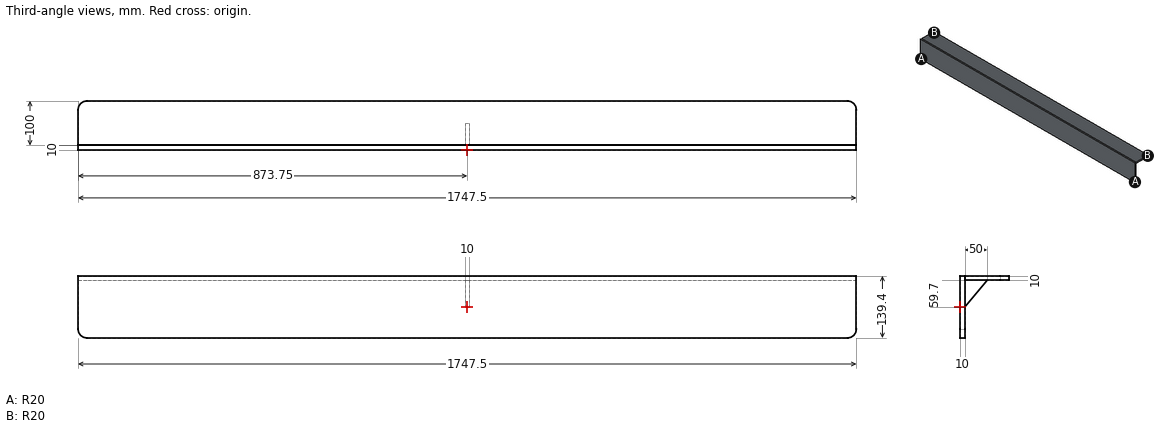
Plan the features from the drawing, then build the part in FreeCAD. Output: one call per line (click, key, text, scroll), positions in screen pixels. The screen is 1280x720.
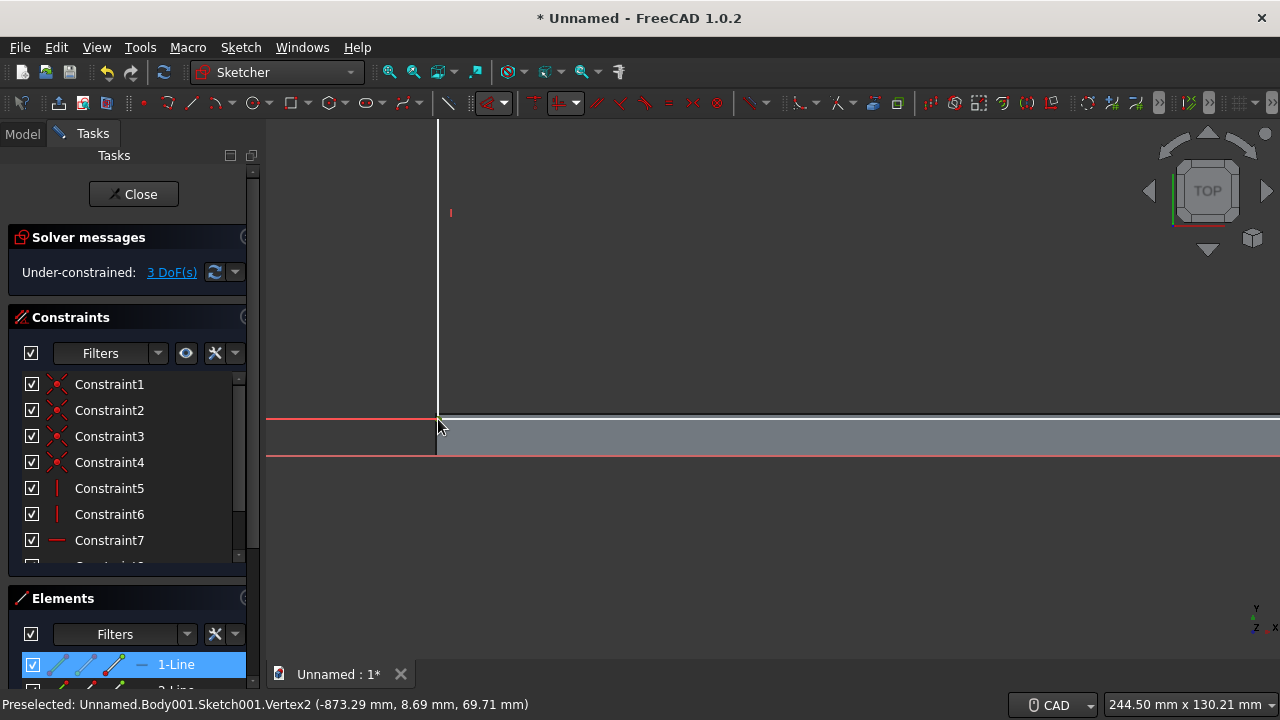
key(i)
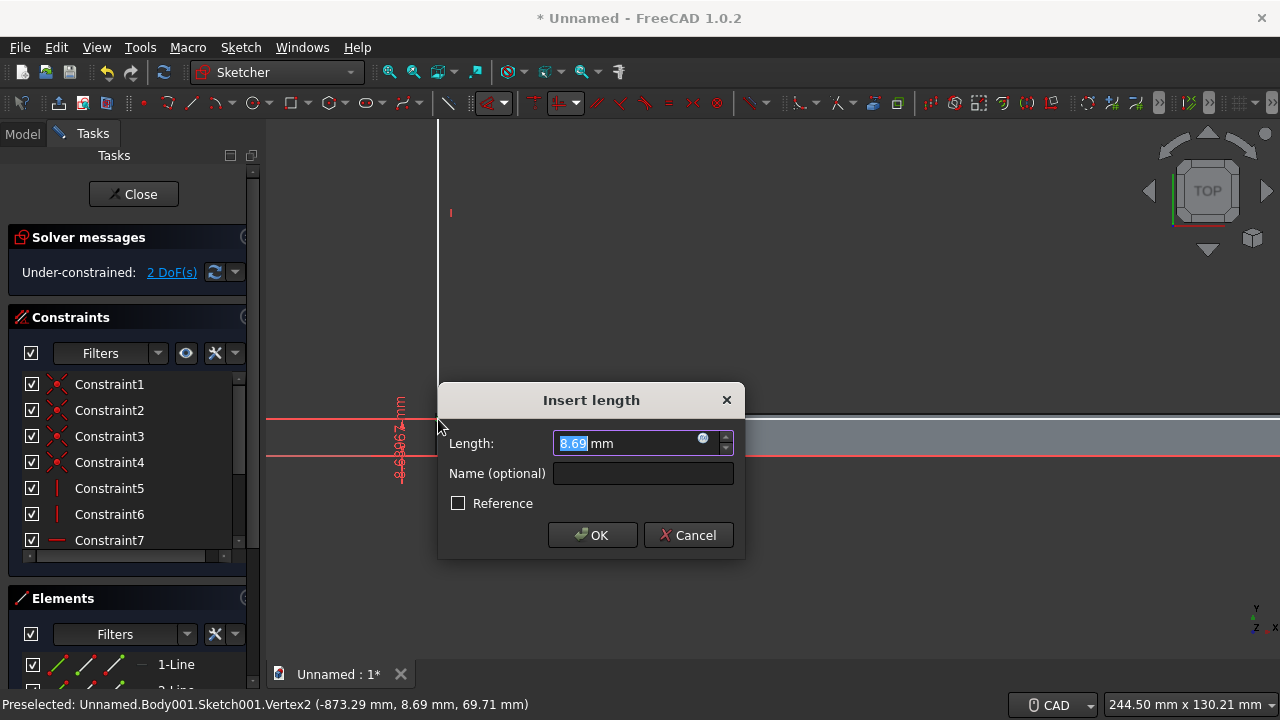
text(10)
key(Return)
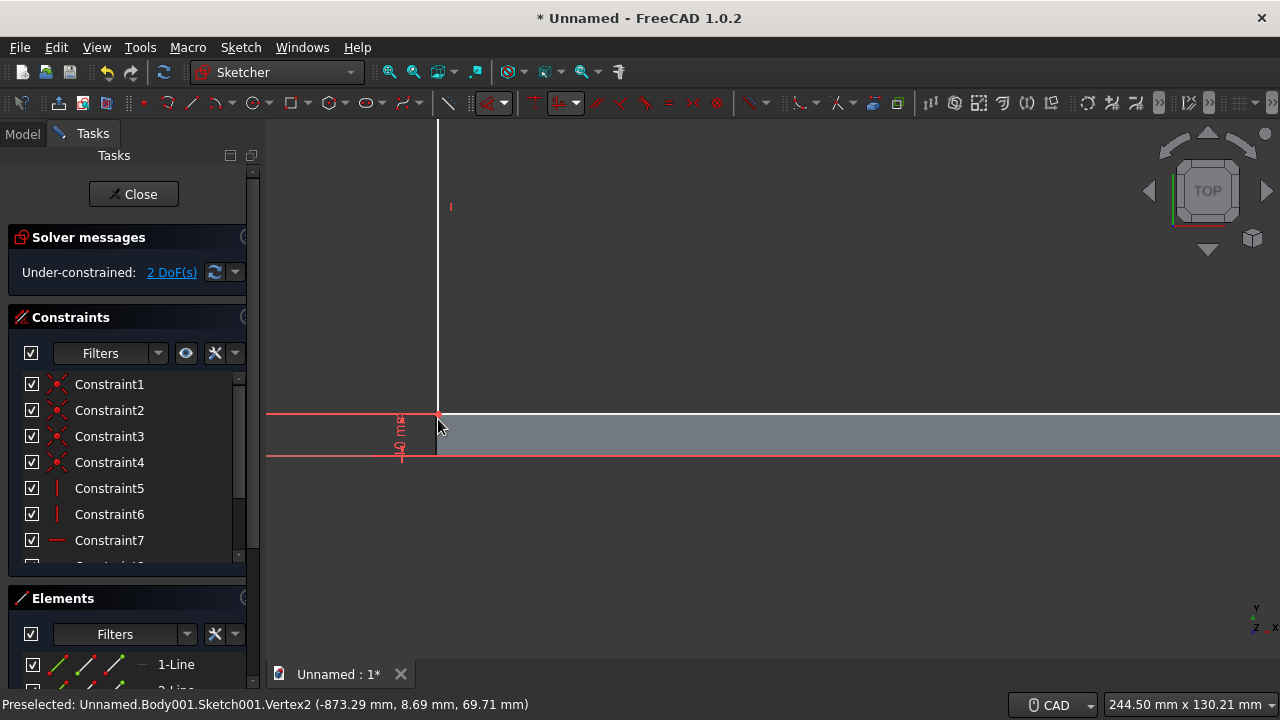
scroll(435, 402, down, 13)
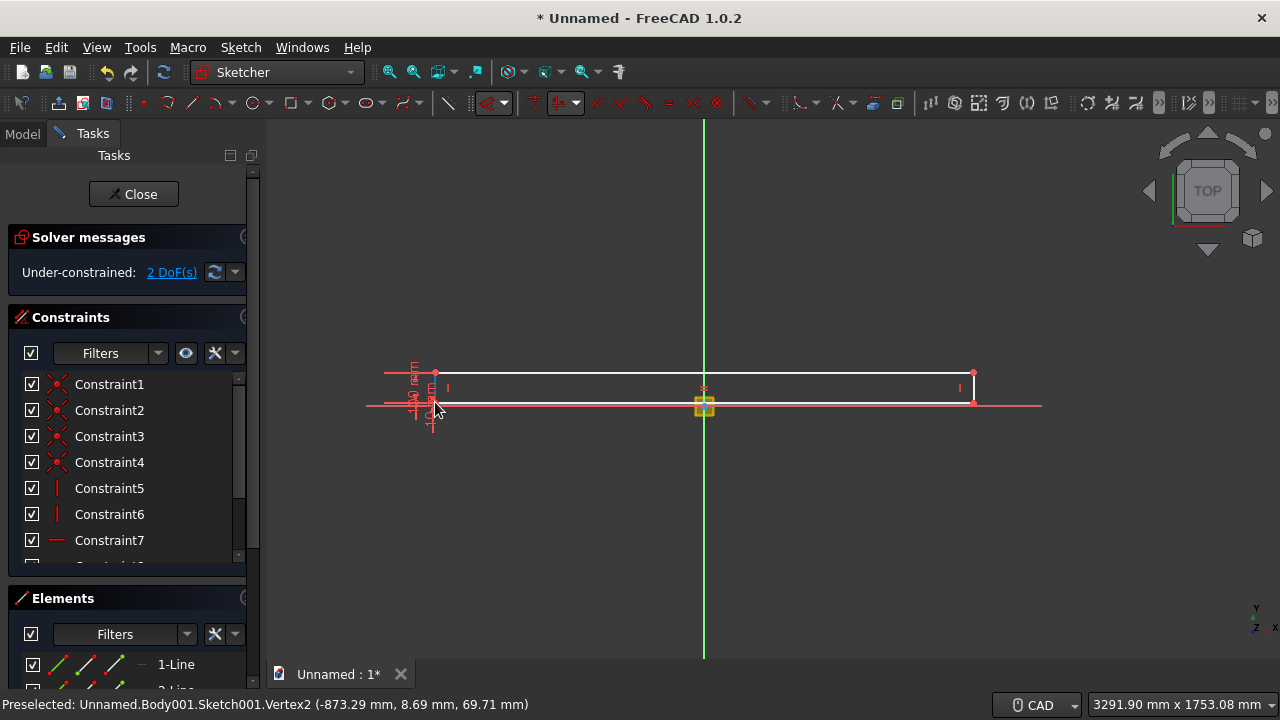
scroll(597, 403, up, 8)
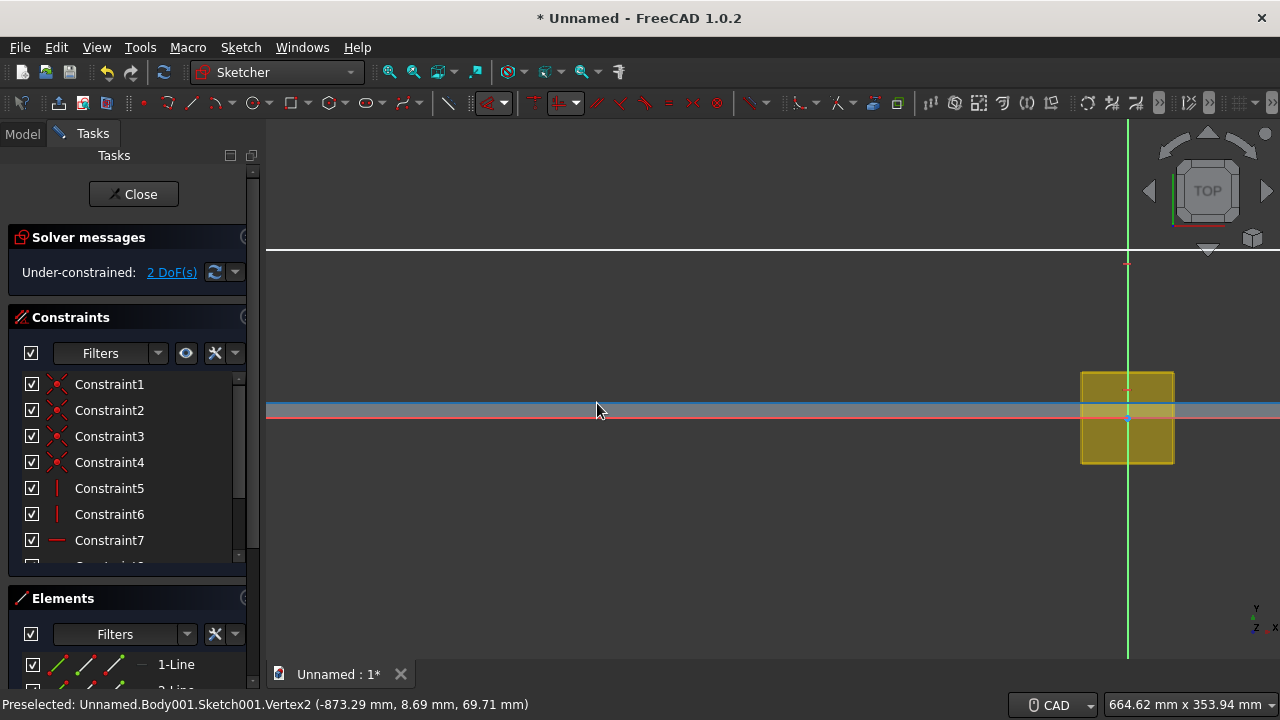
click(595, 403)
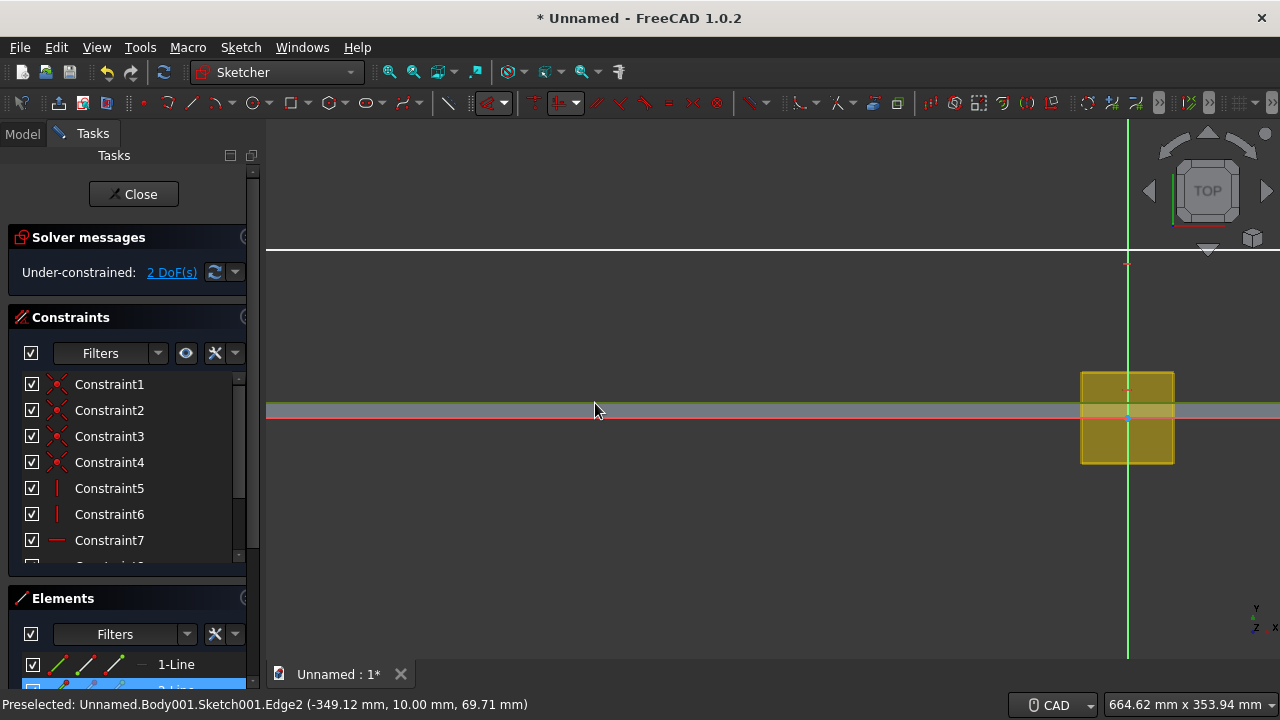
key(l)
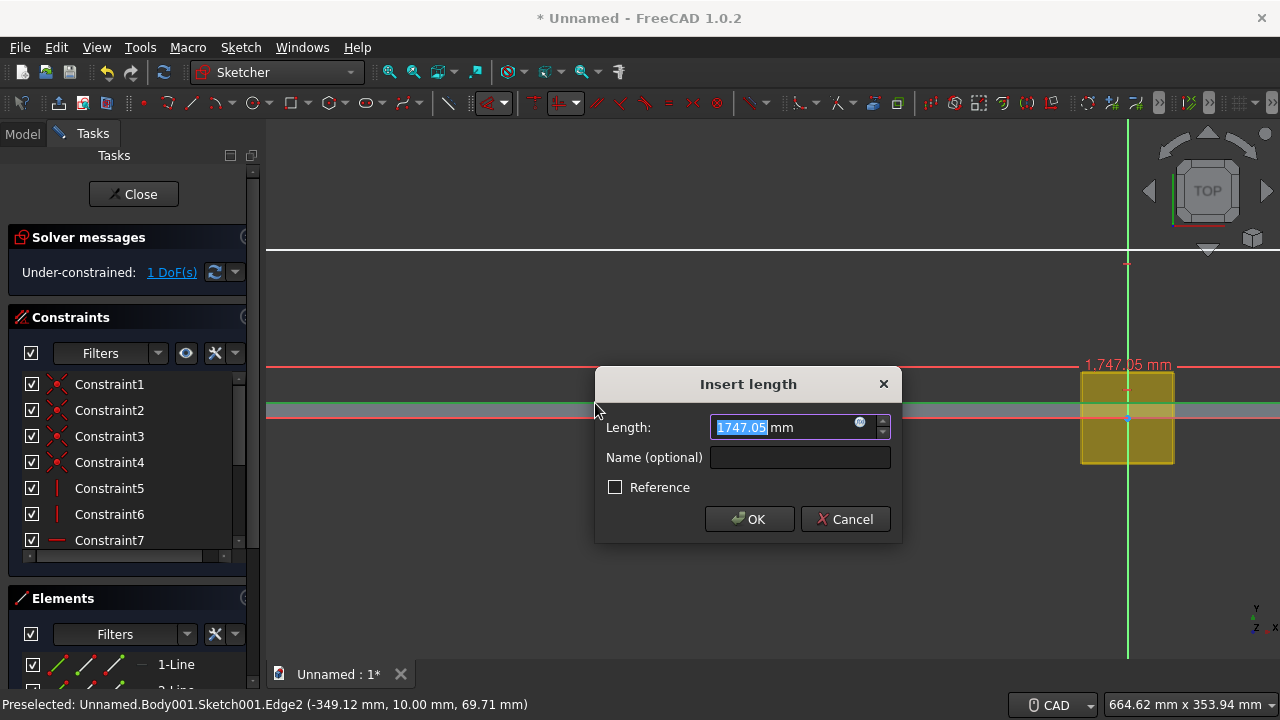
text(1747.5)
key(Return)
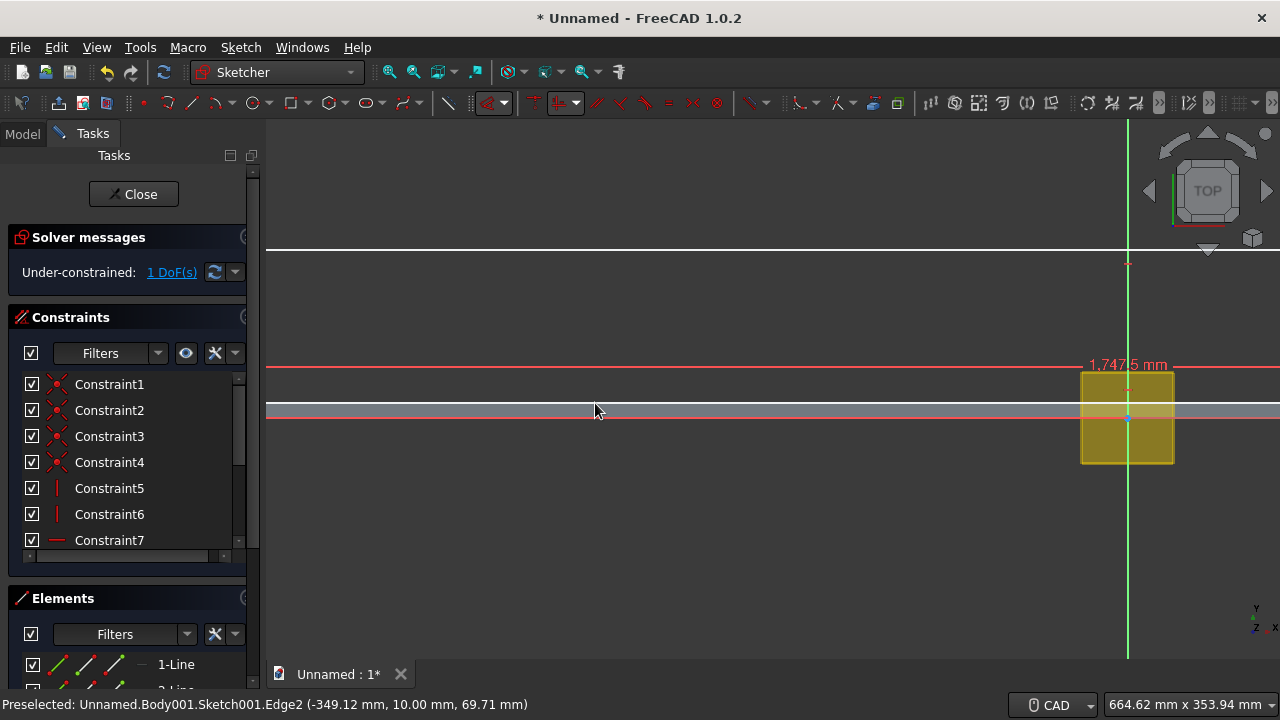
scroll(597, 403, down, 8)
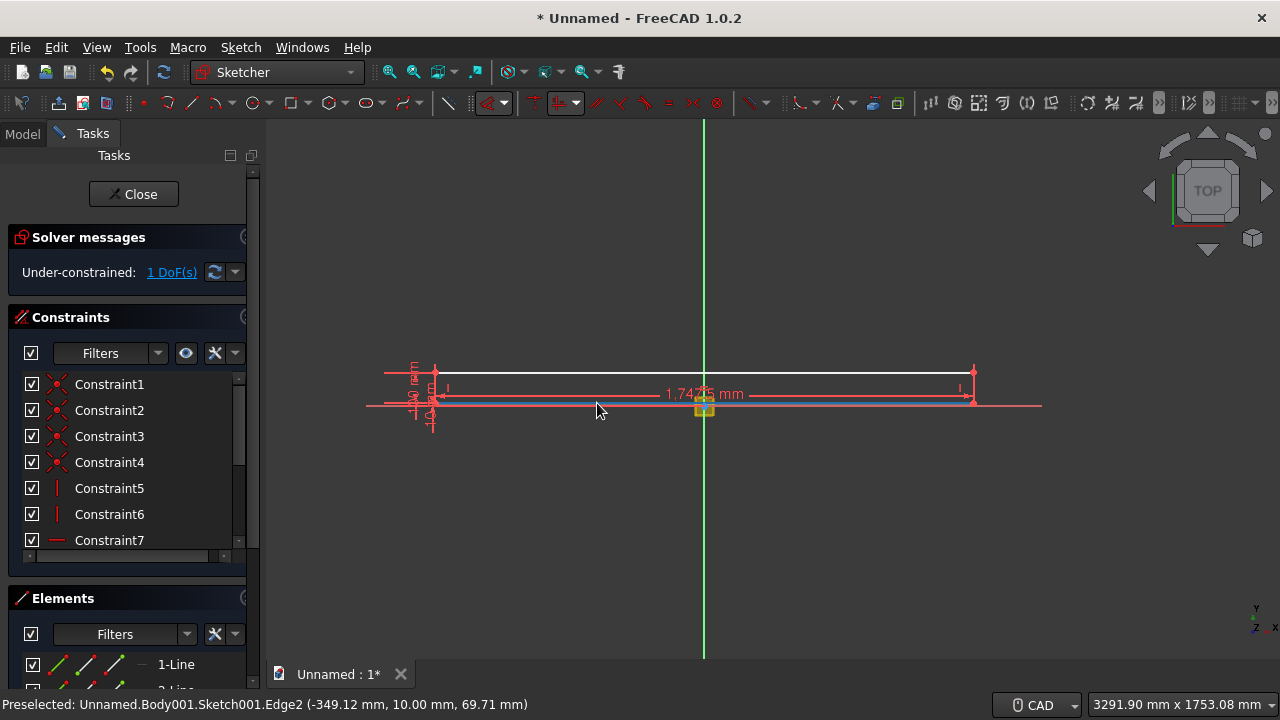
click(435, 373)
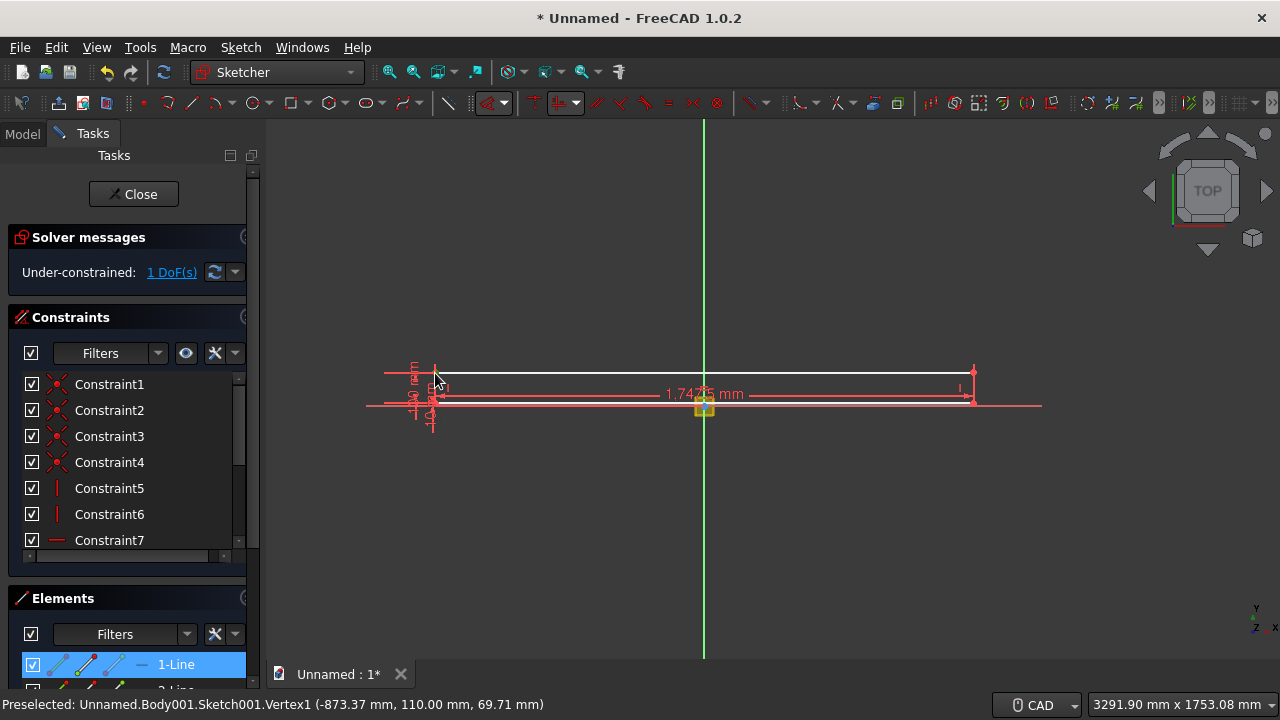
click(506, 104)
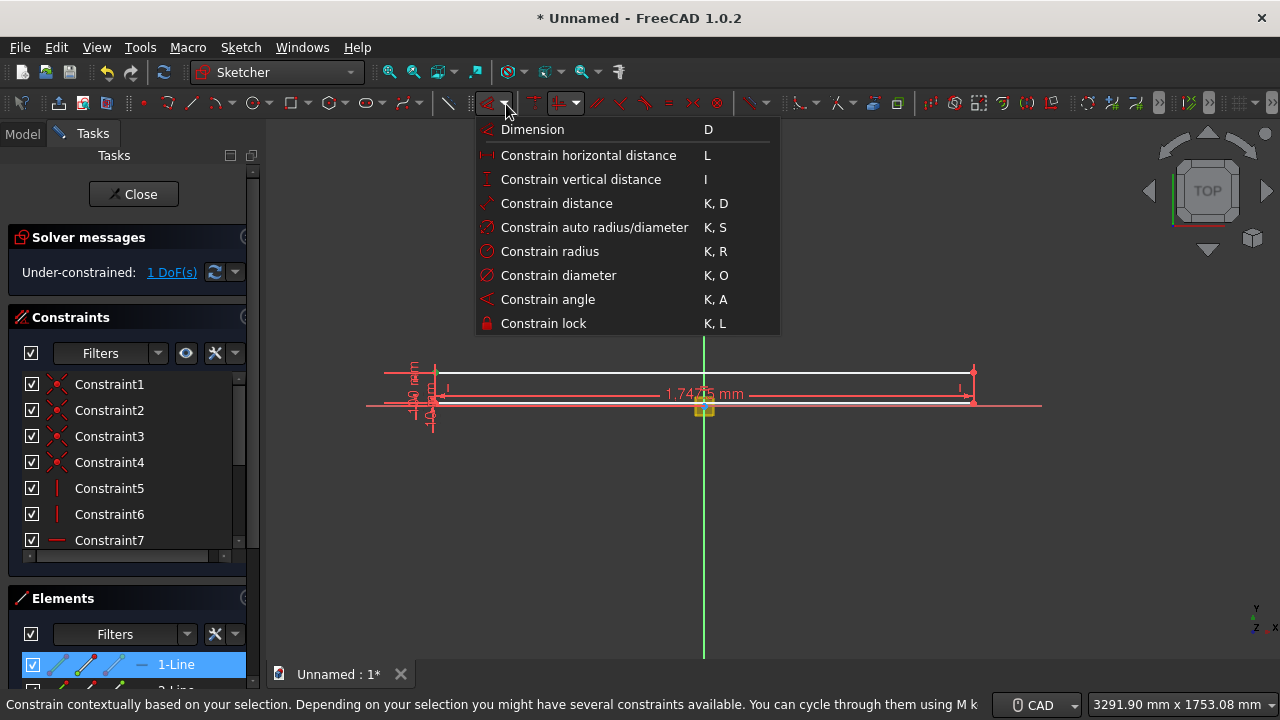
click(628, 155)